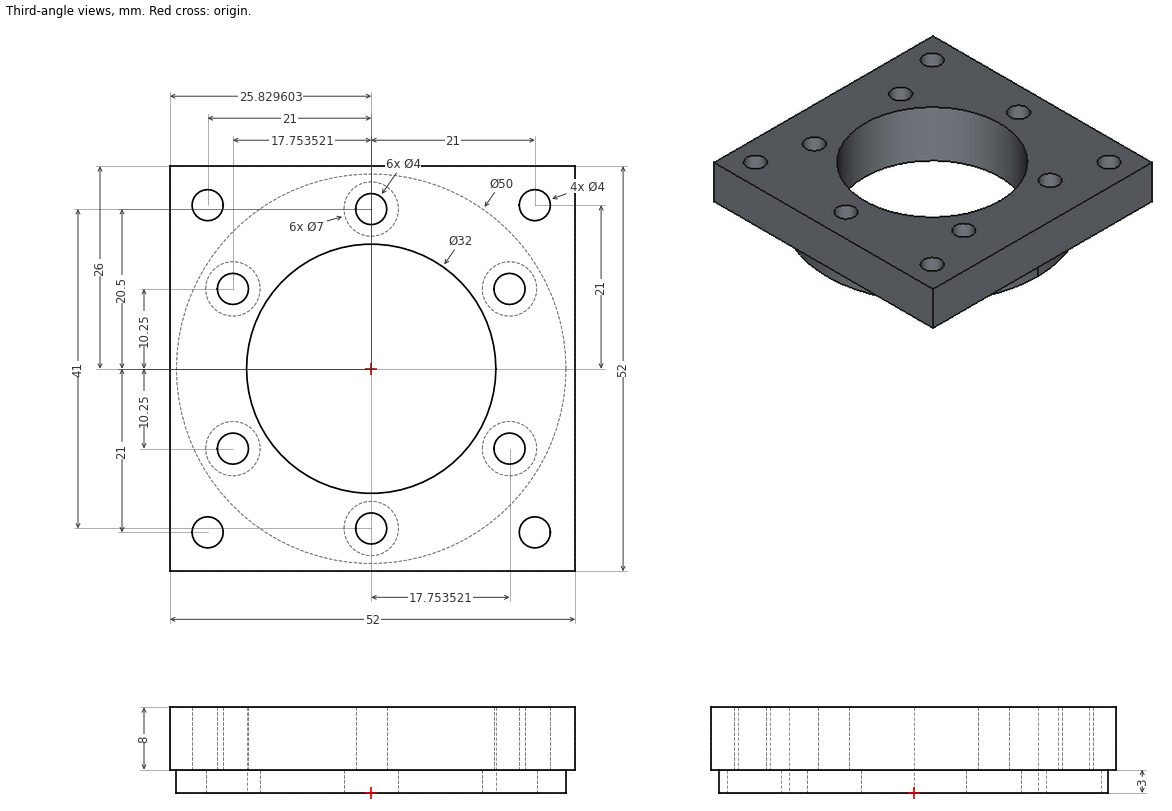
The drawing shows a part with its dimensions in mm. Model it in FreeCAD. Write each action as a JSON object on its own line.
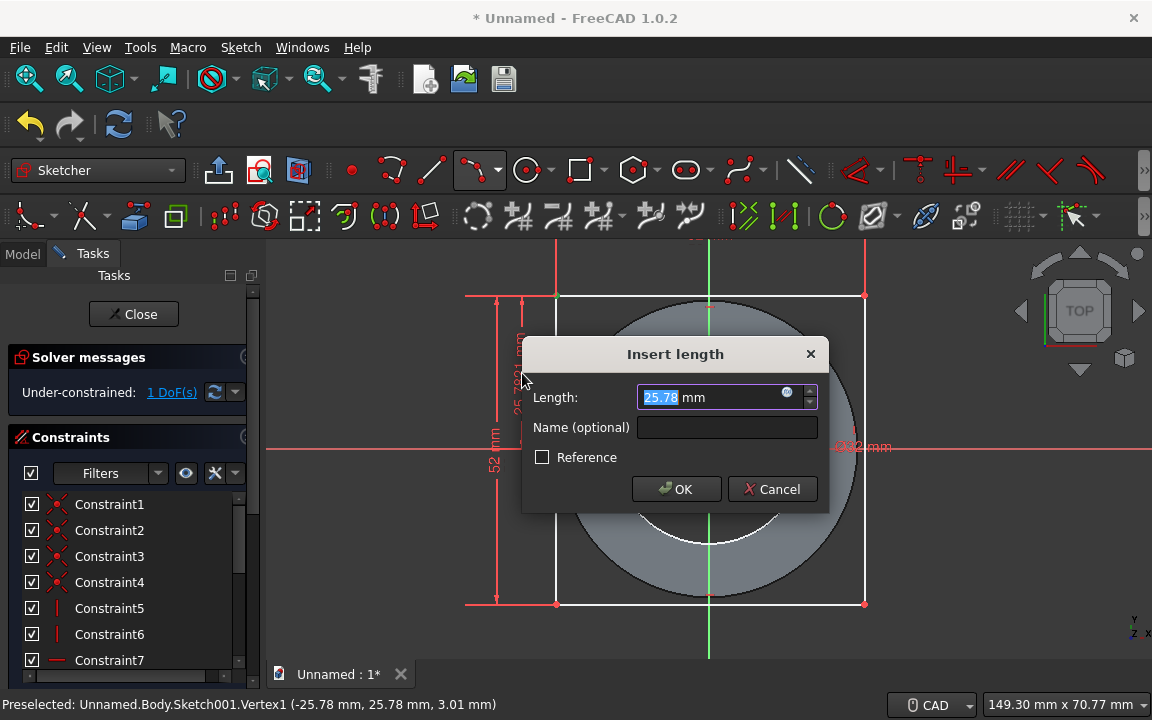
{"action": "type", "text": "26"}
{"action": "key", "text": "Return"}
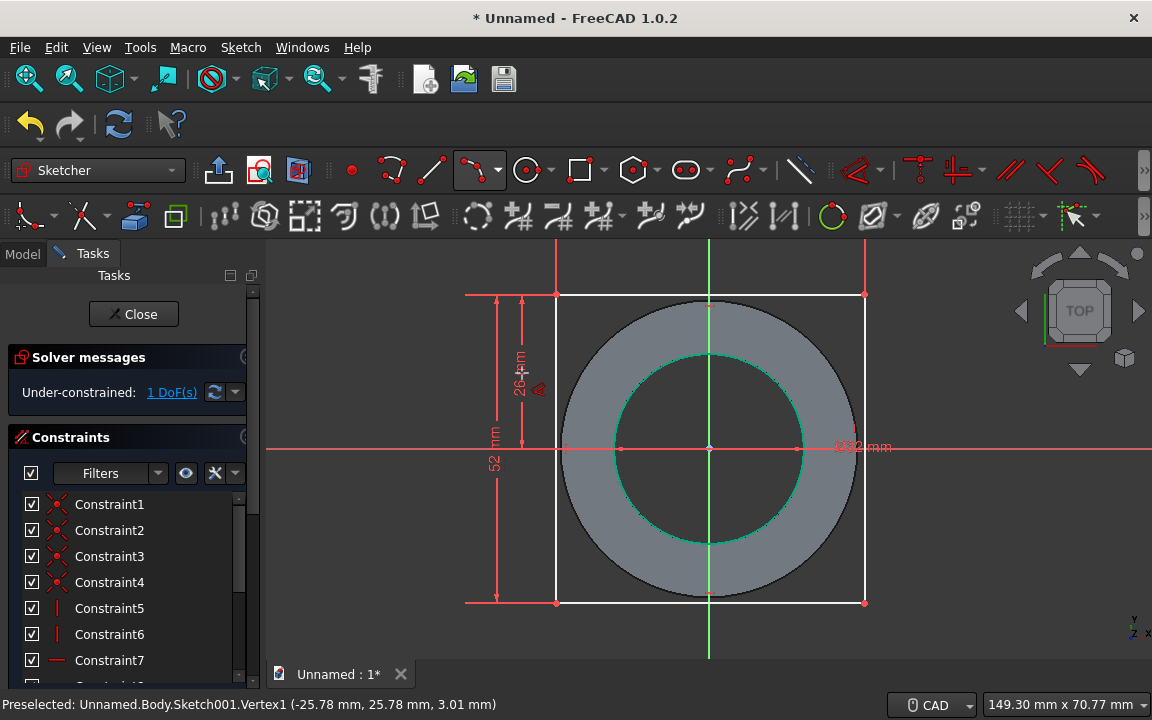
{"action": "left_click", "coordinate": [556, 295]}
{"action": "left_click", "coordinate": [597, 483]}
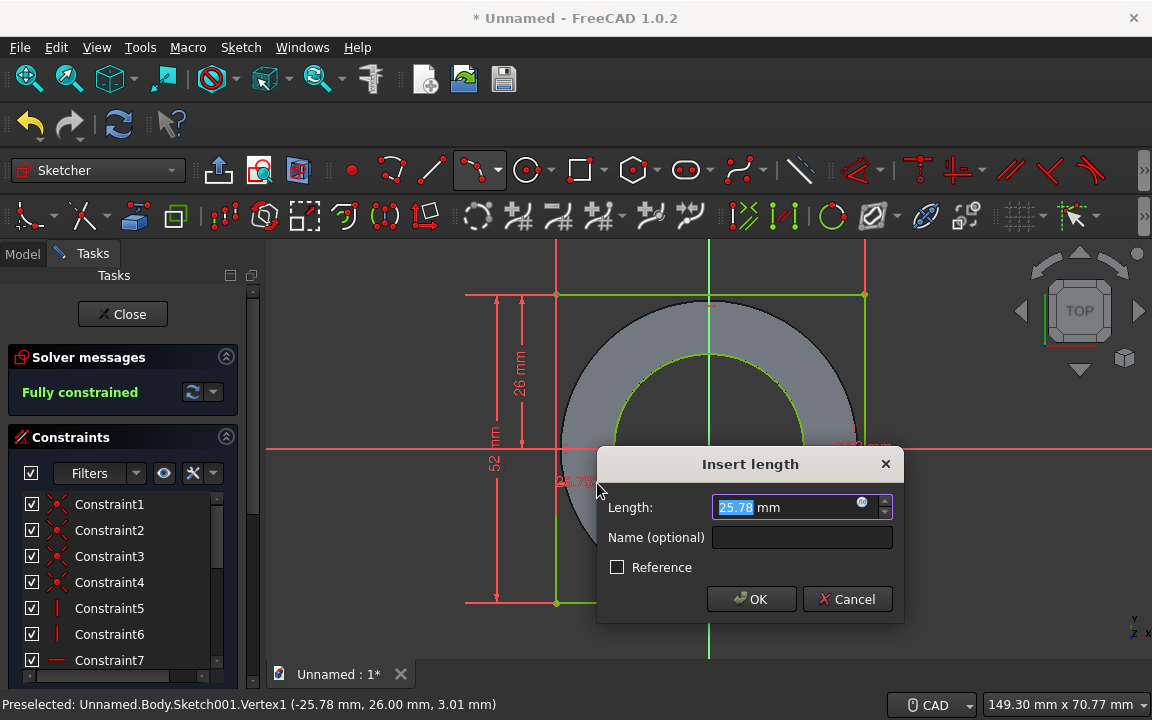
{"action": "type", "text": "25.829603"}
{"action": "key", "text": "Return"}
{"action": "key", "text": "Escape"}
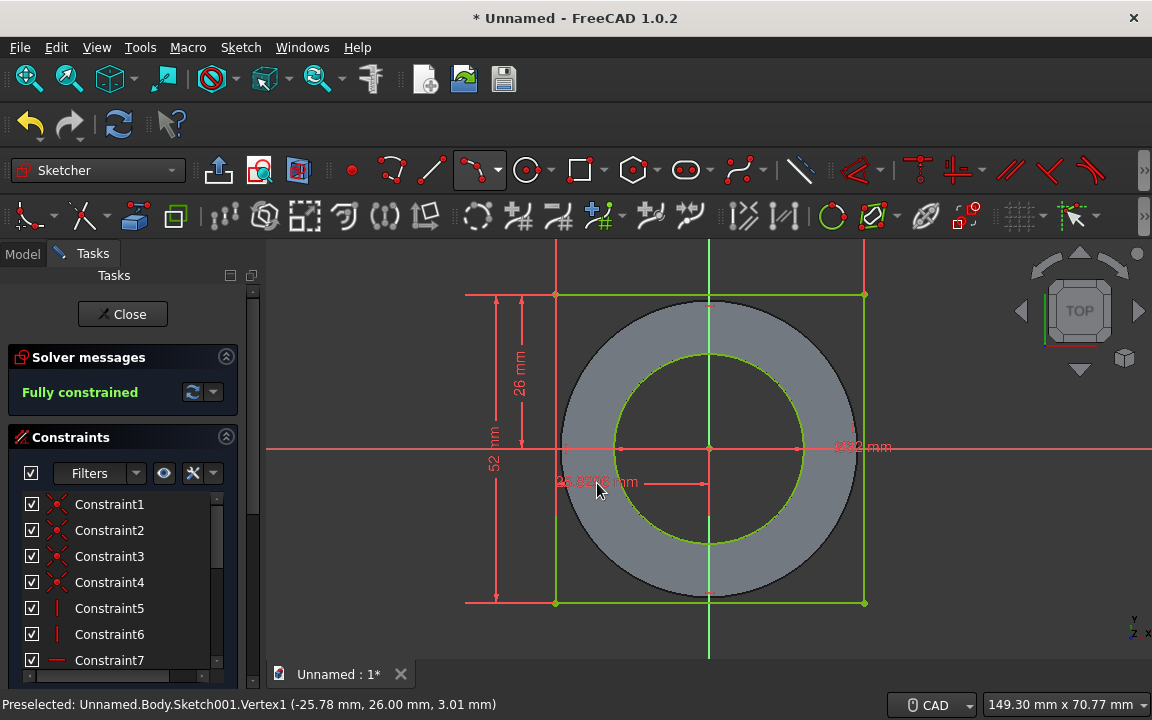
{"action": "left_click", "coordinate": [123, 314]}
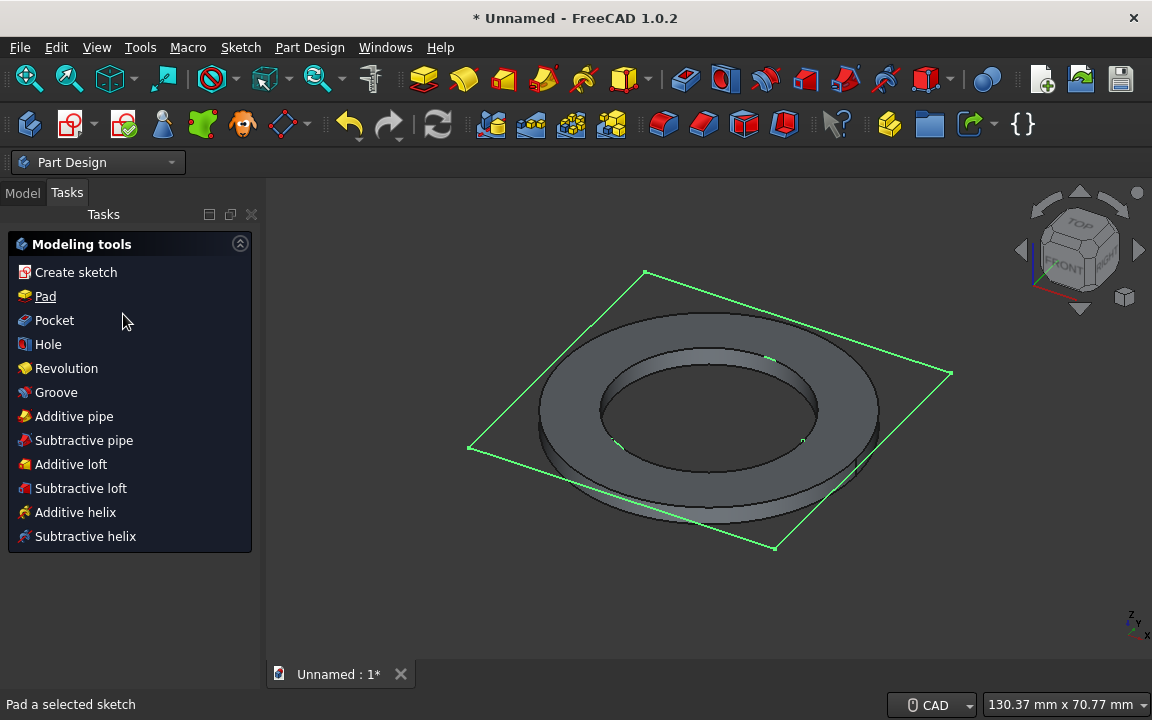
{"action": "left_click", "coordinate": [424, 80]}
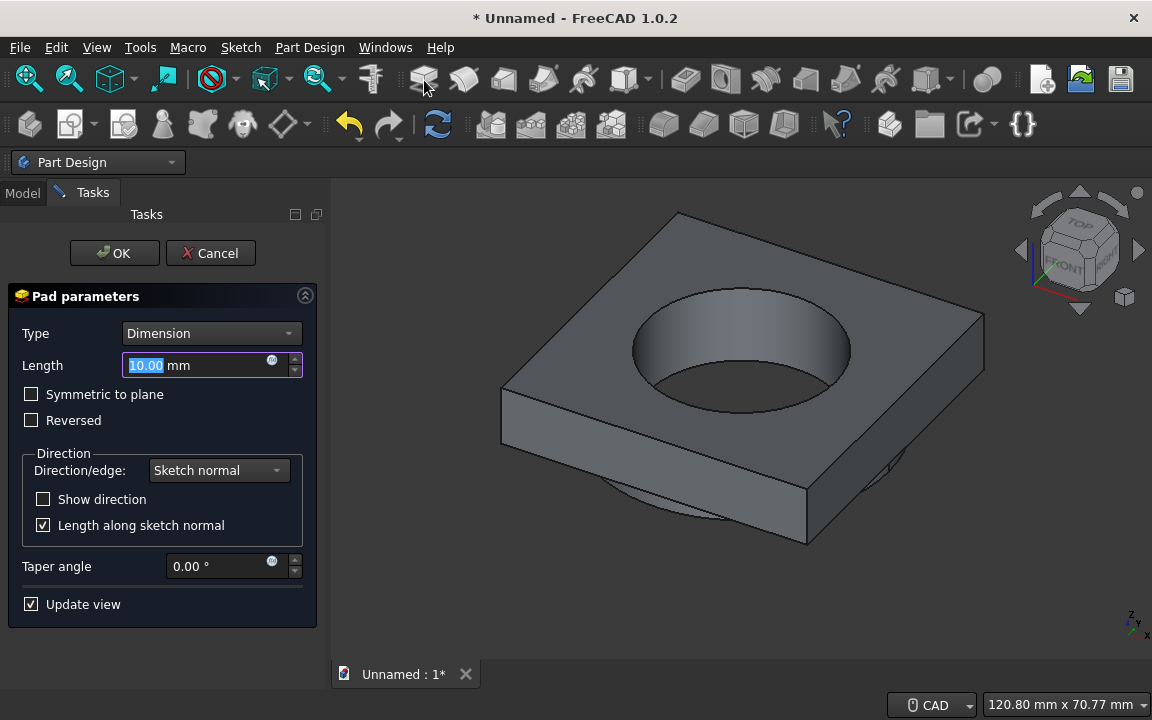
{"action": "type", "text": "8"}
{"action": "key", "text": "Tab"}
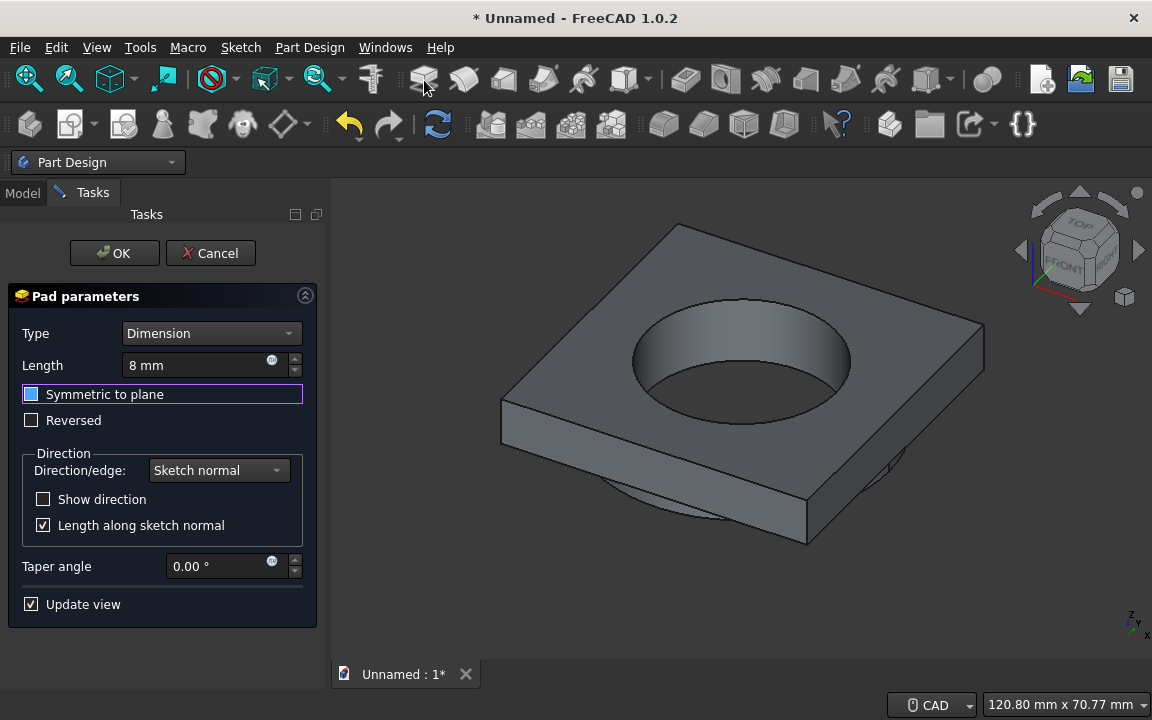
{"action": "left_click", "coordinate": [115, 253]}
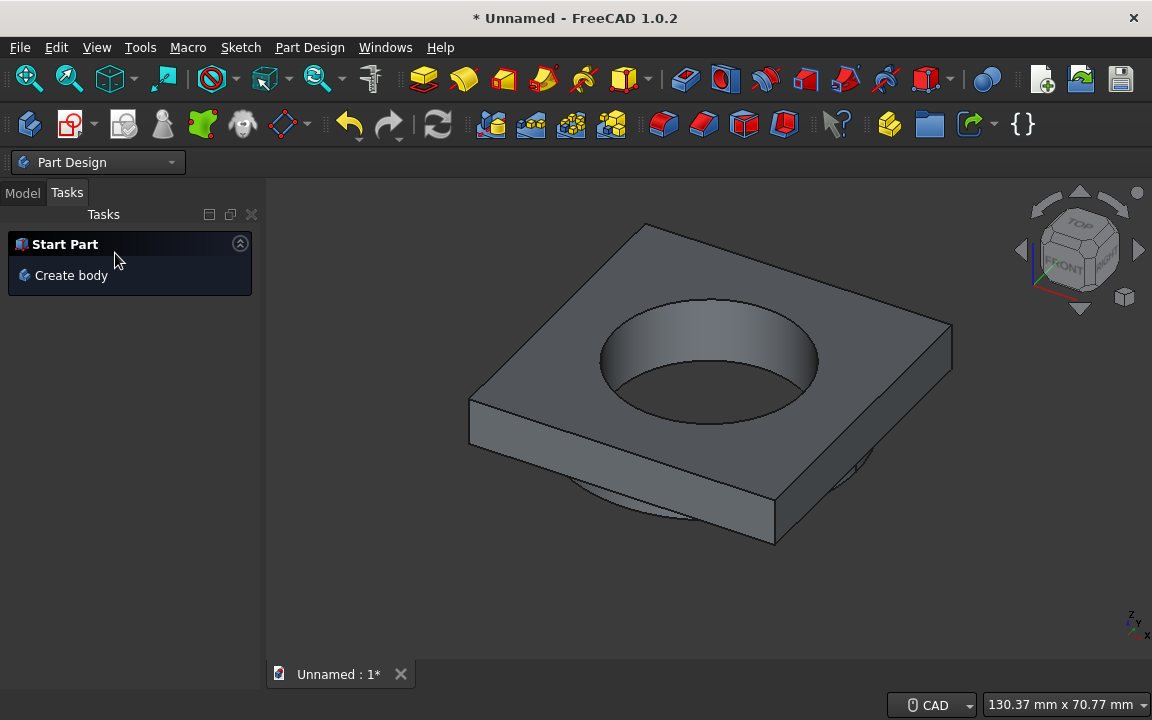
{"action": "key", "text": "5"}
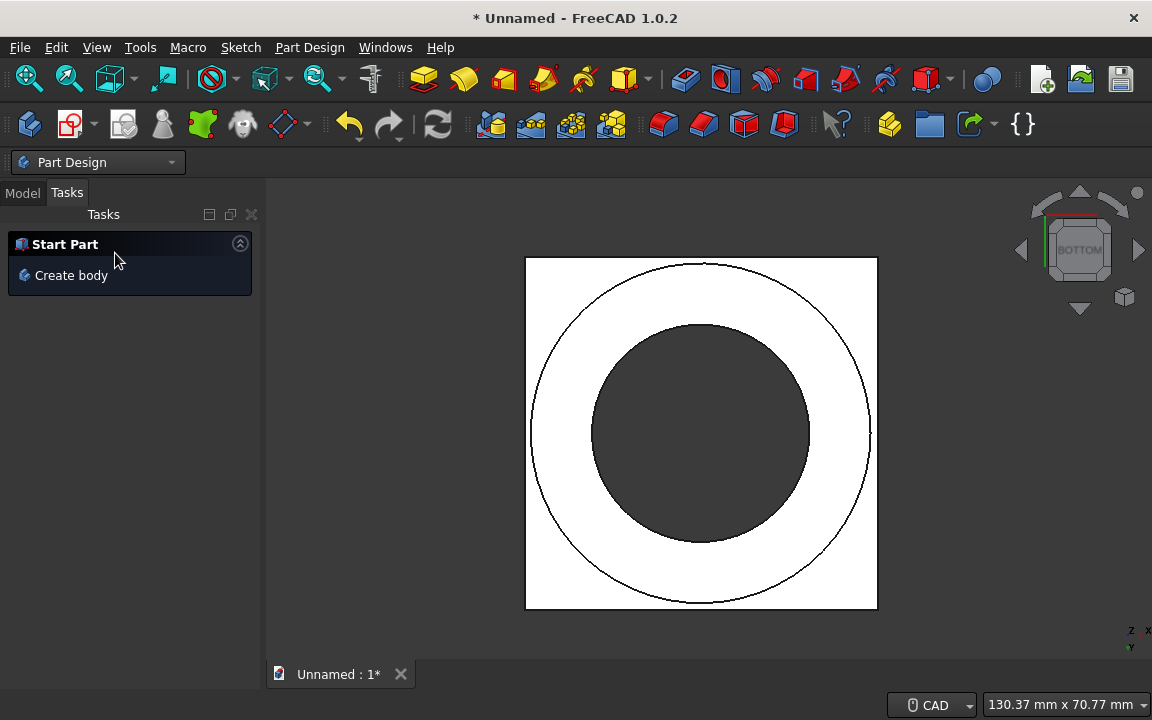
{"action": "left_click", "coordinate": [604, 529]}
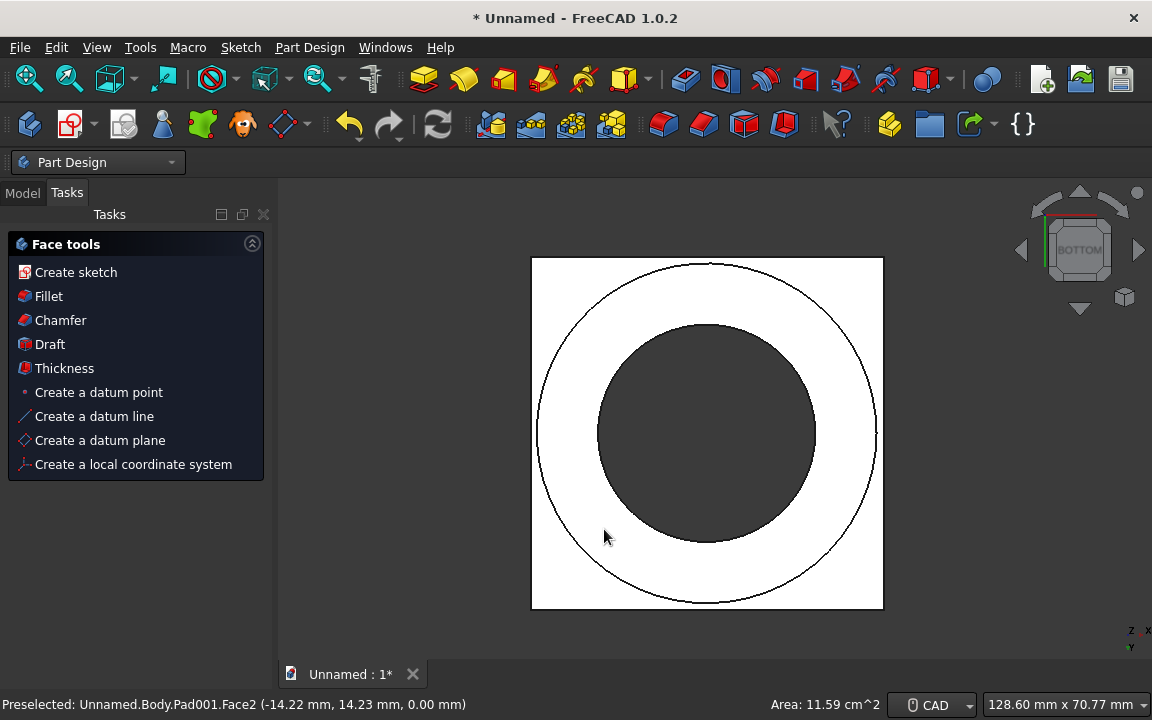
{"action": "left_click", "coordinate": [70, 124]}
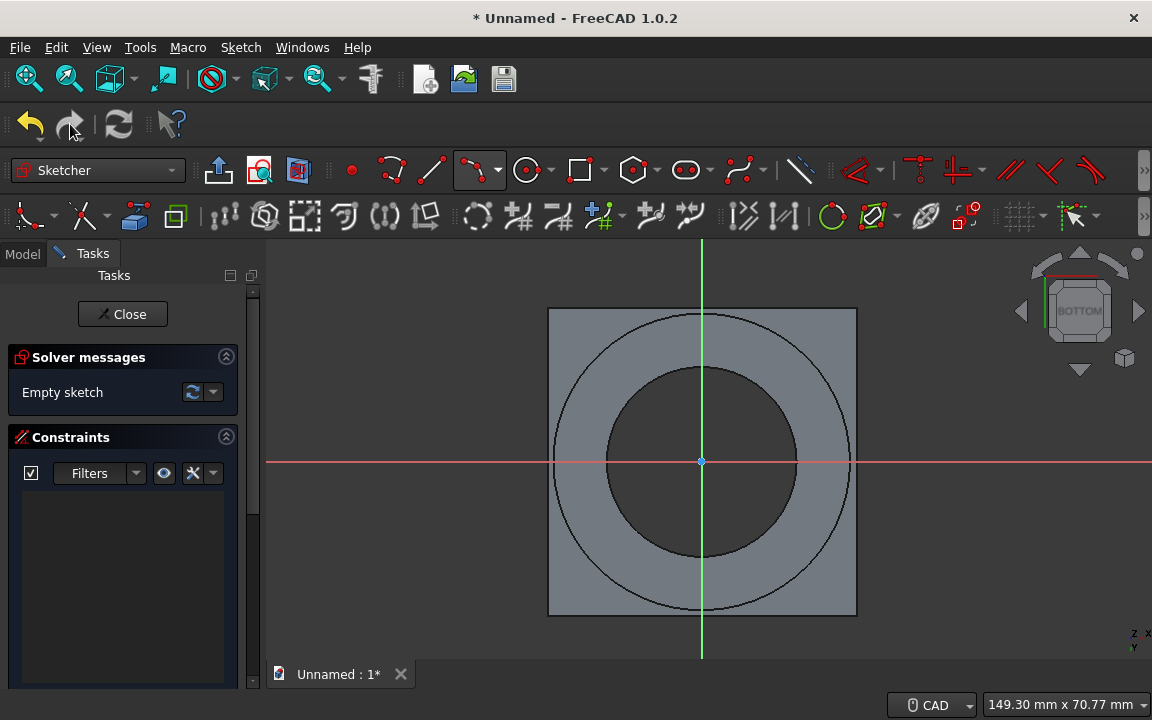
{"action": "key", "text": "g c"}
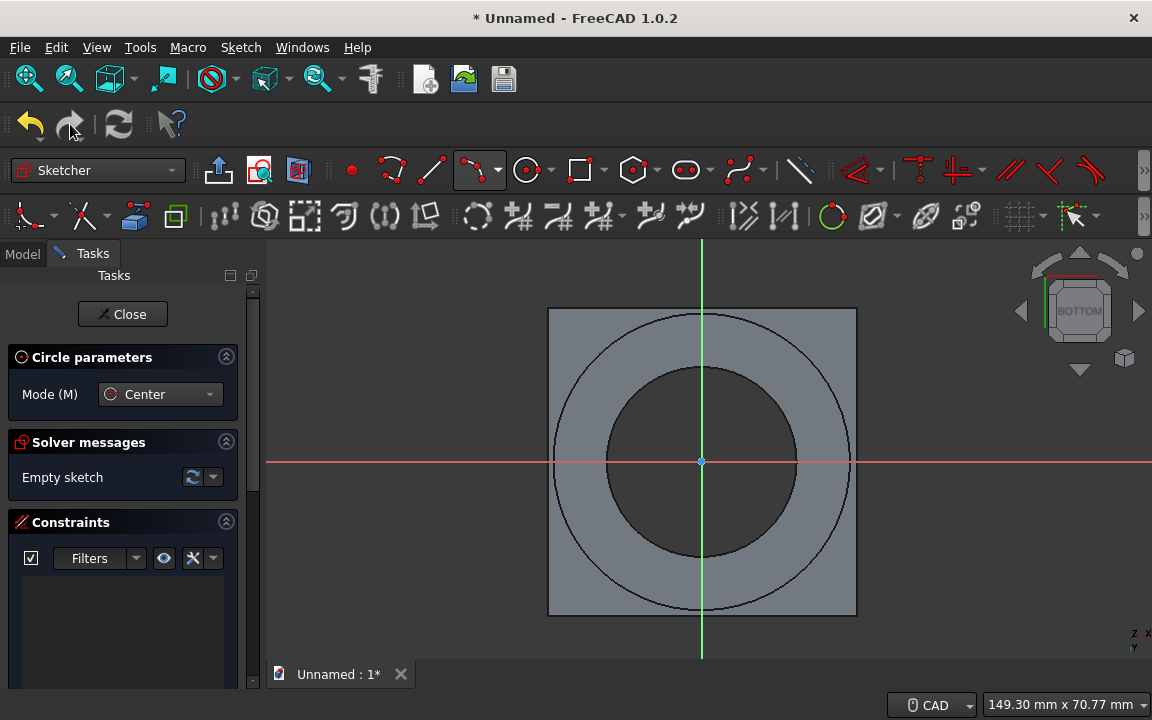
{"action": "scroll", "coordinate": [702, 584], "scroll_direction": "up", "scroll_amount": 4}